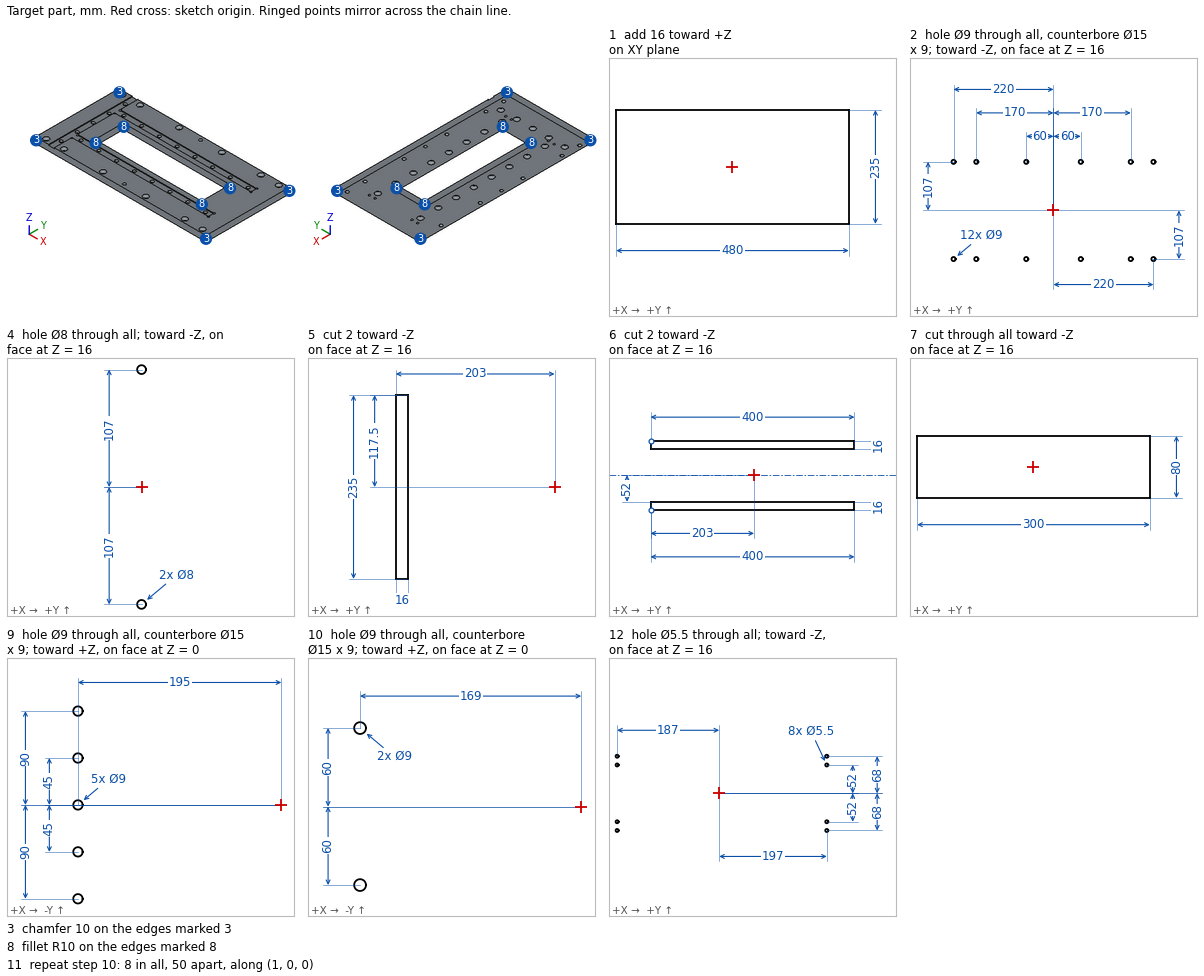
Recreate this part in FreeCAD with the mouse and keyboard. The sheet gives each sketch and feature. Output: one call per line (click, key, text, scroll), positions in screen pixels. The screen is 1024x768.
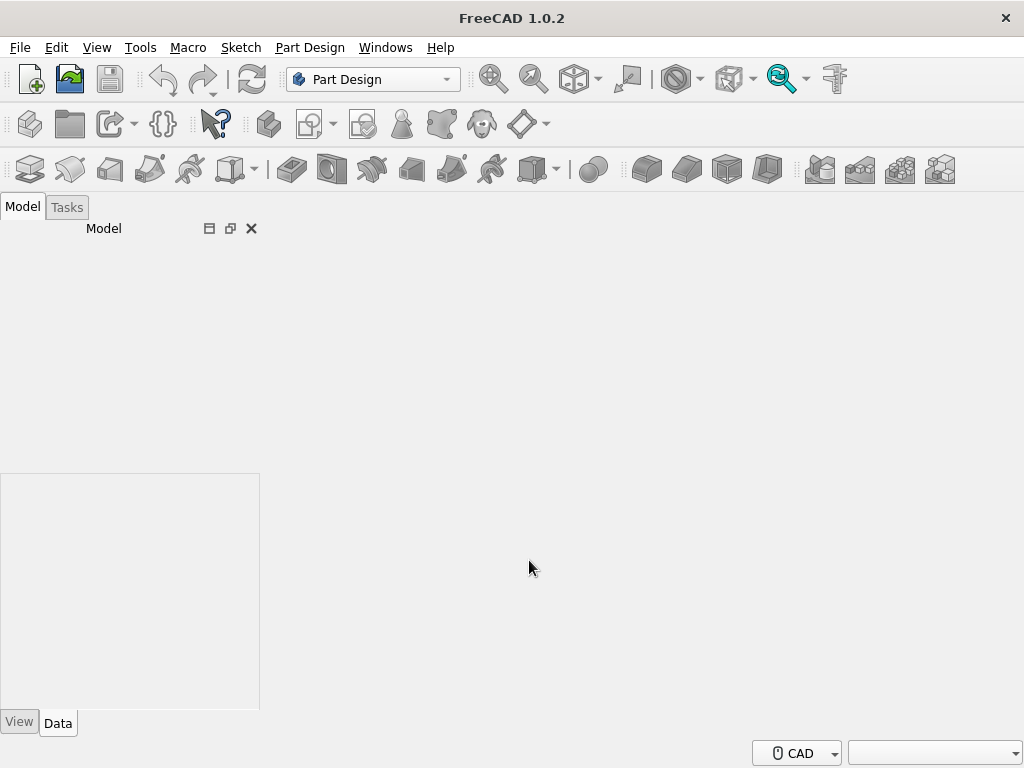
click(30, 80)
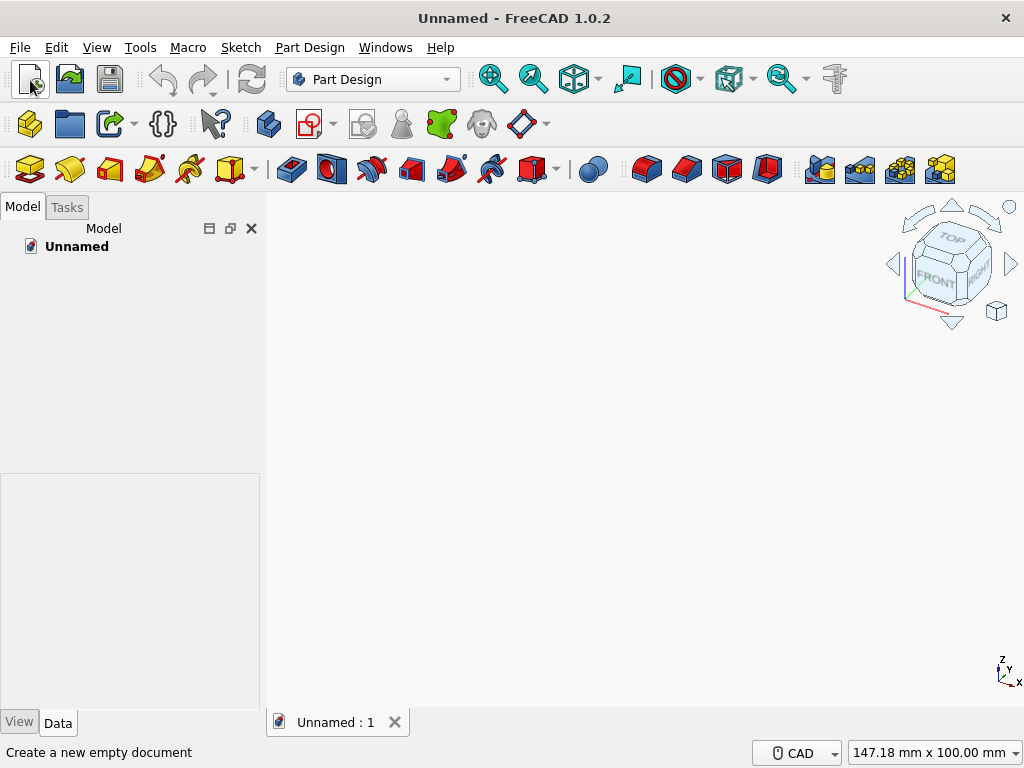
click(310, 124)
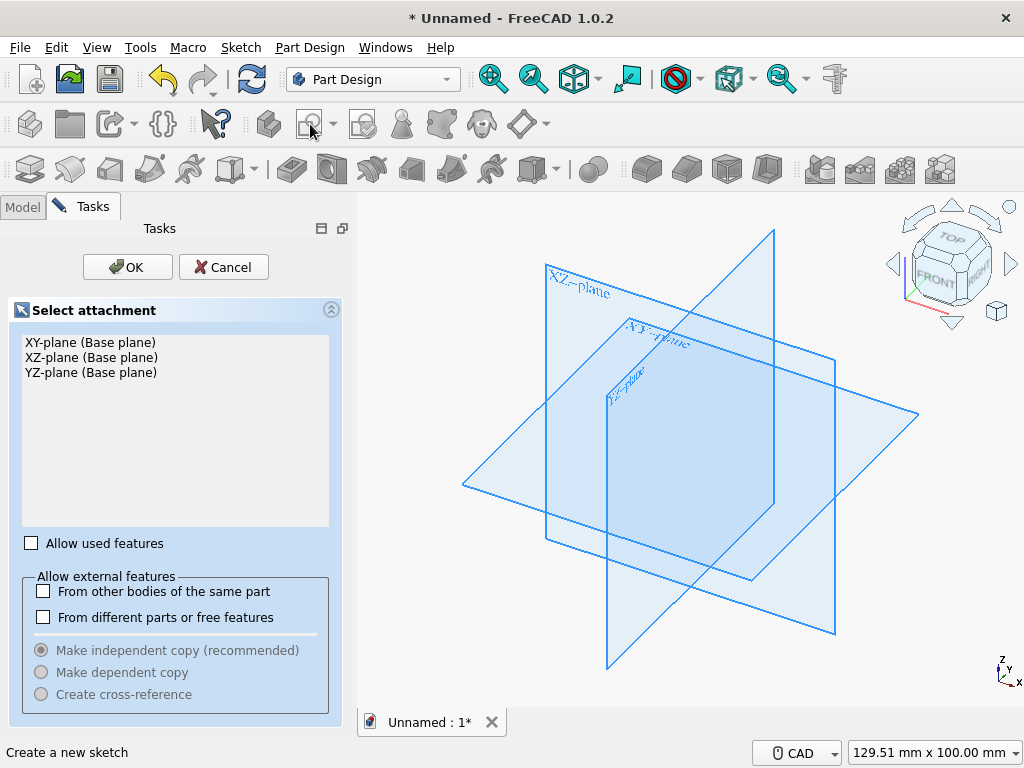
click(82, 342)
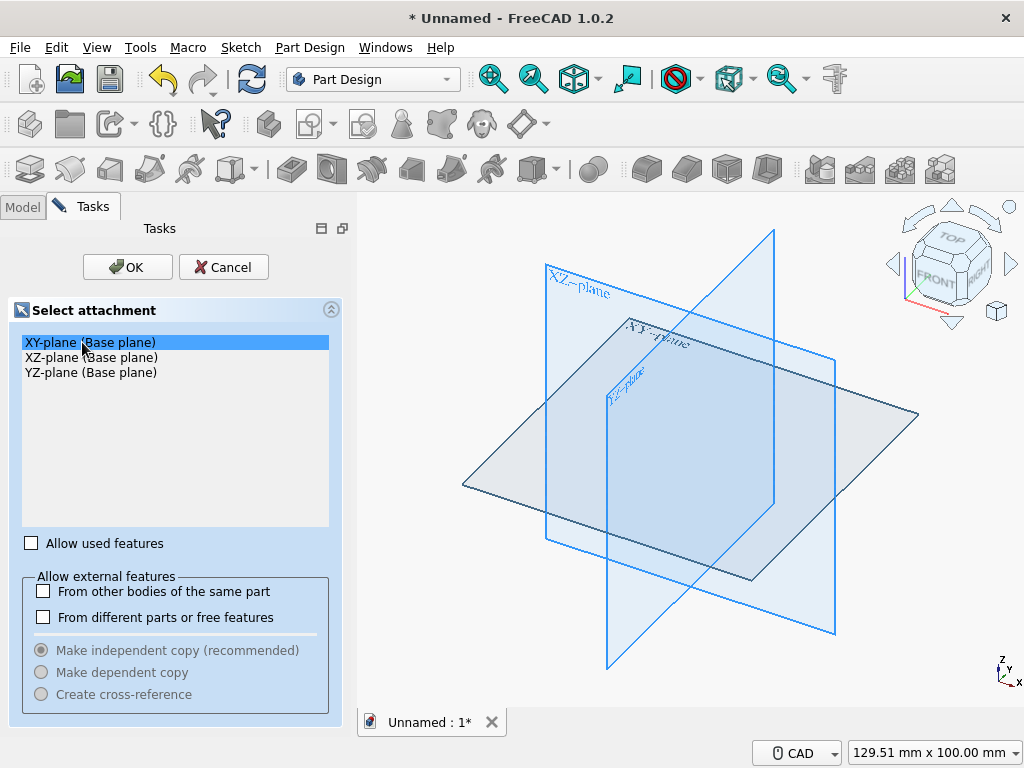
click(128, 267)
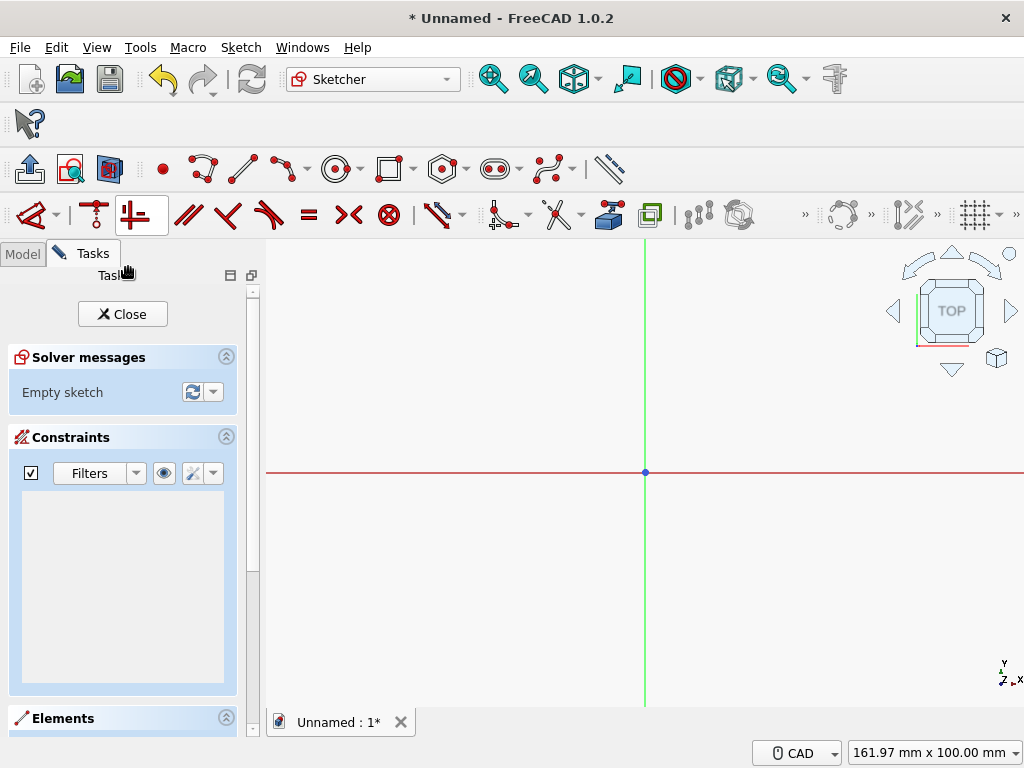
scroll(563, 473, down, 9)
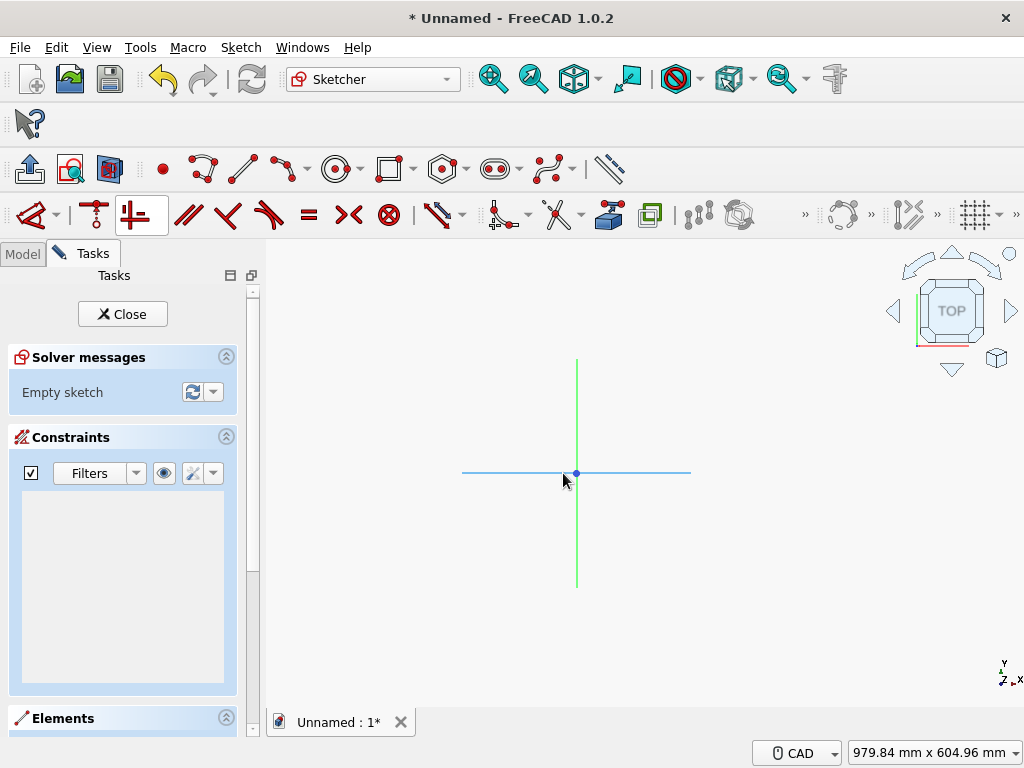
key(g)
key(v)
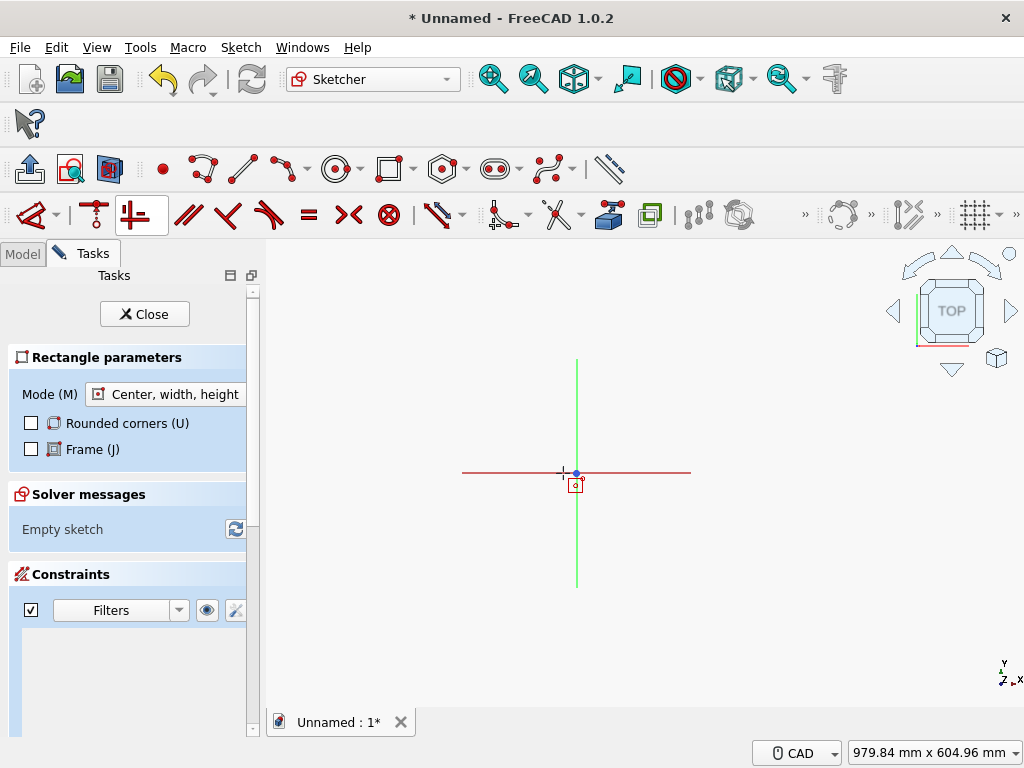
click(577, 473)
move(763, 383)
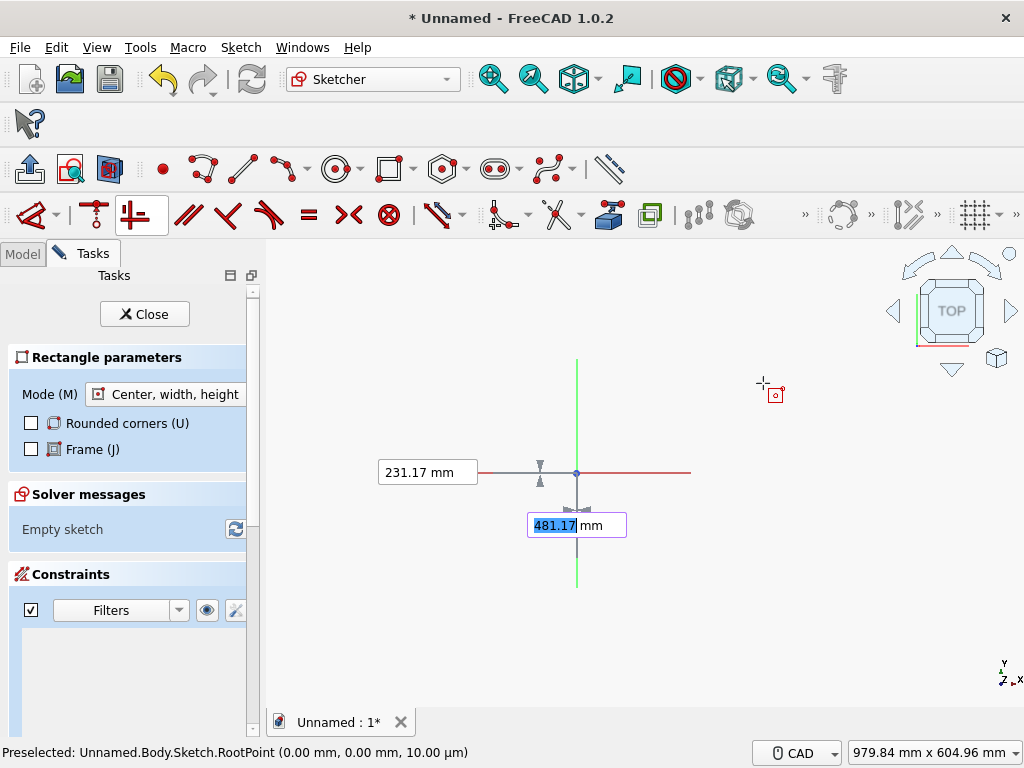
text(480)
key(Tab)
text(235)
key(Return)
key(Escape)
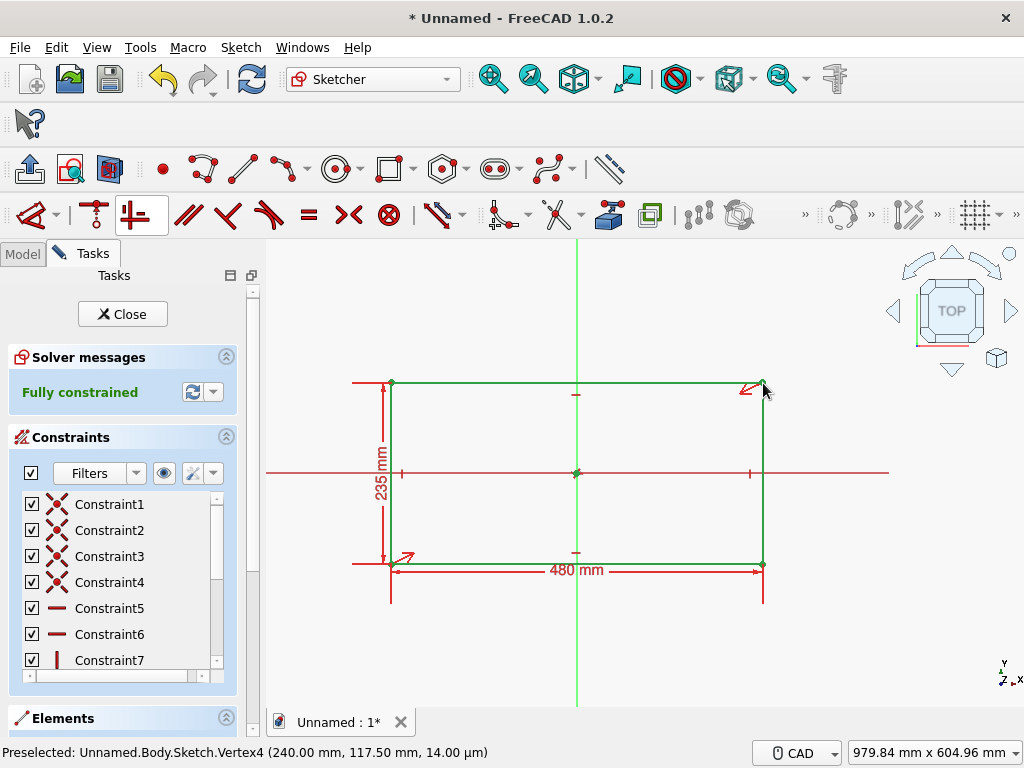
click(123, 314)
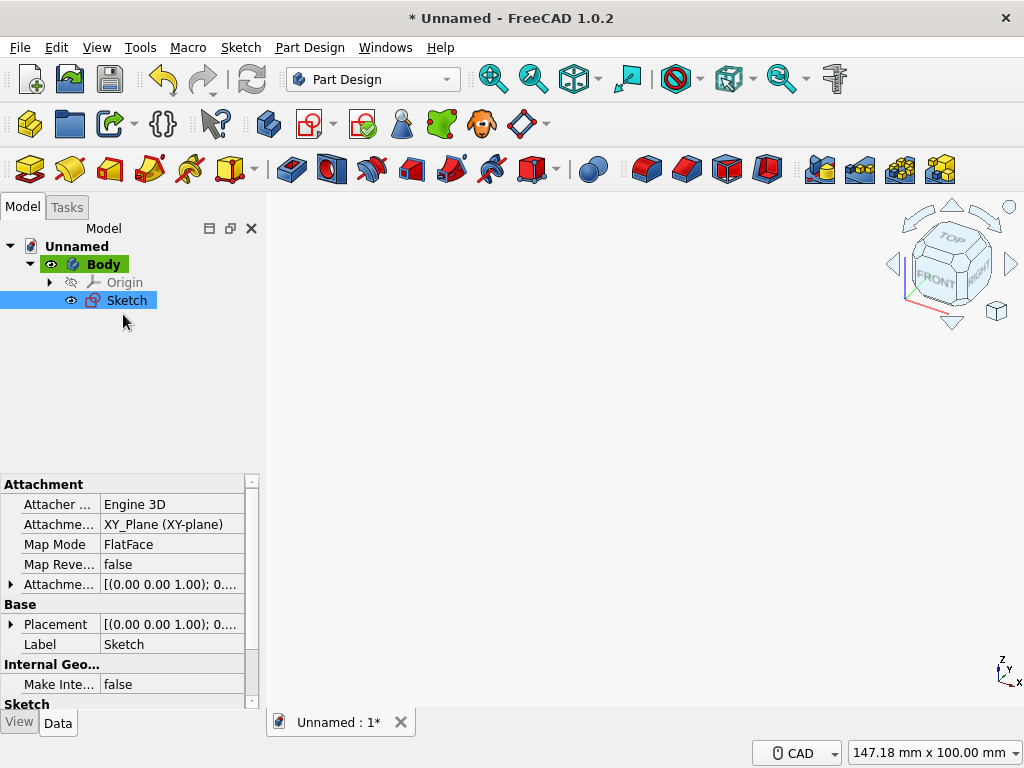
click(30, 170)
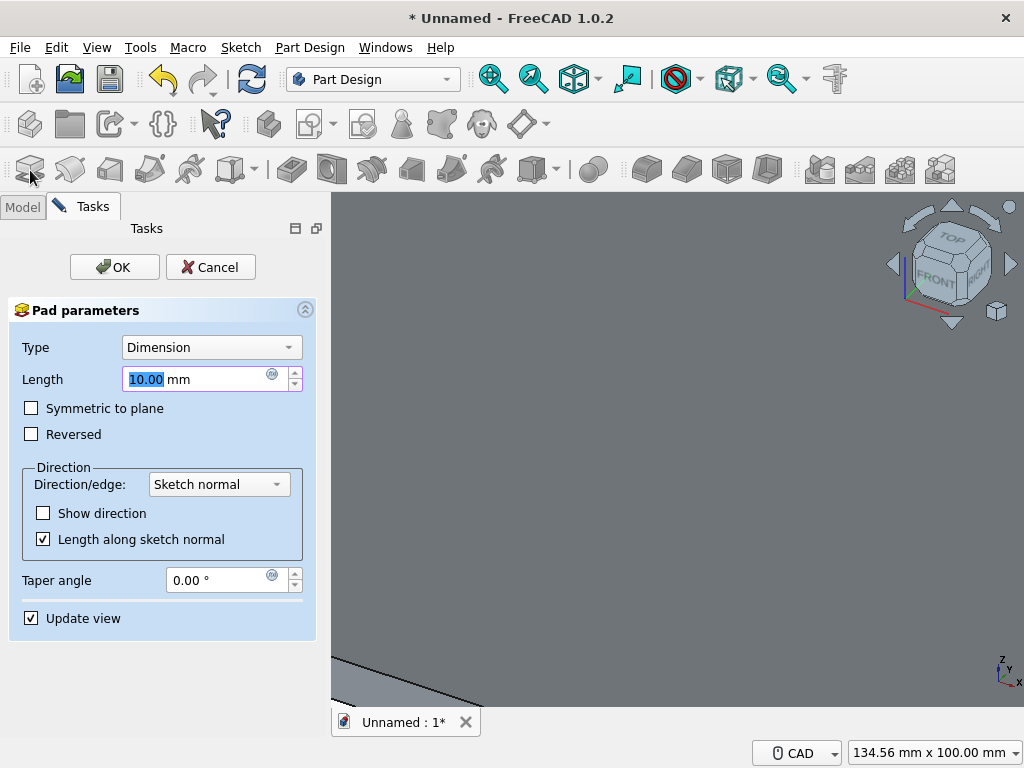
text(16)
key(Tab)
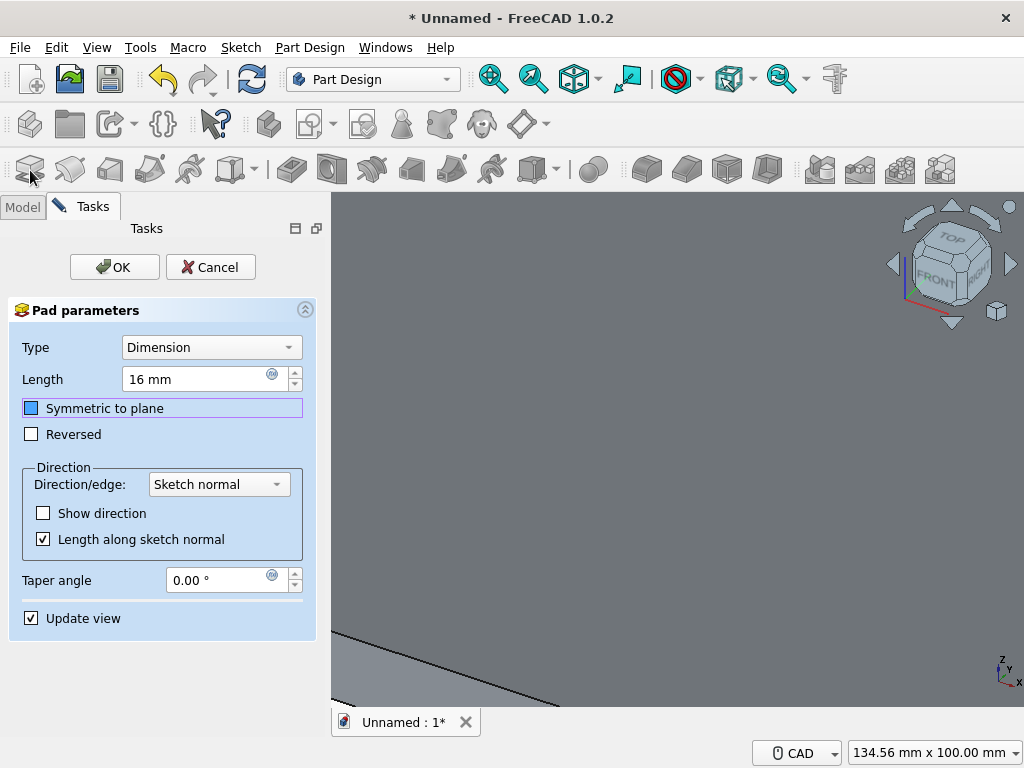
click(115, 267)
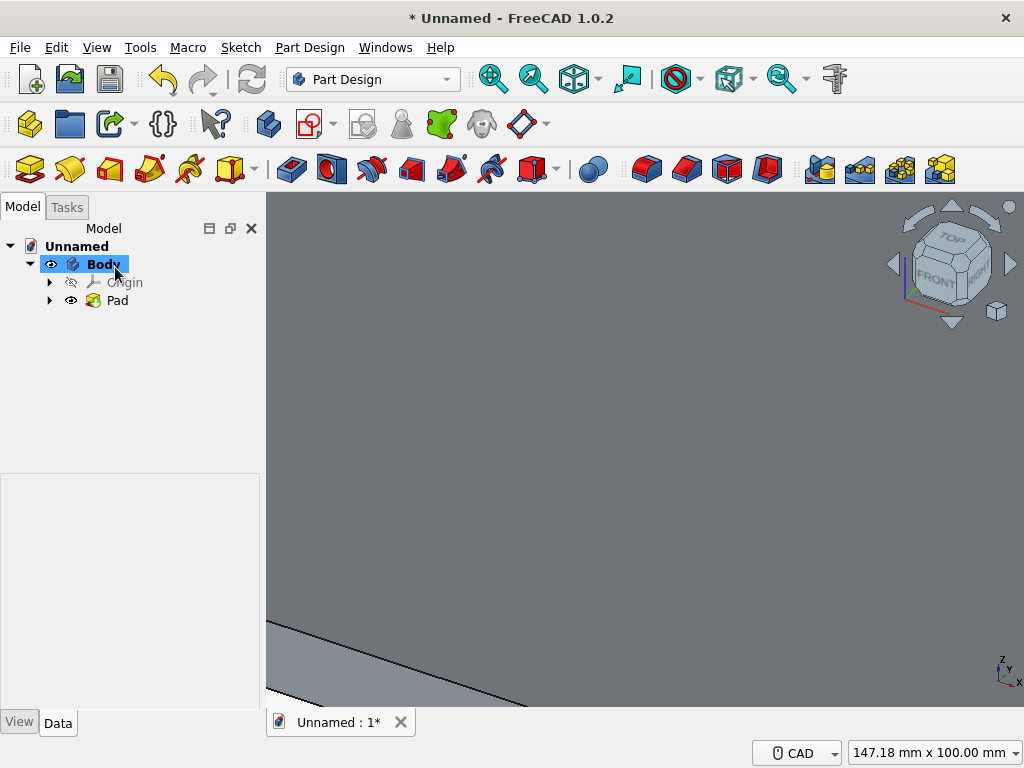
click(494, 80)